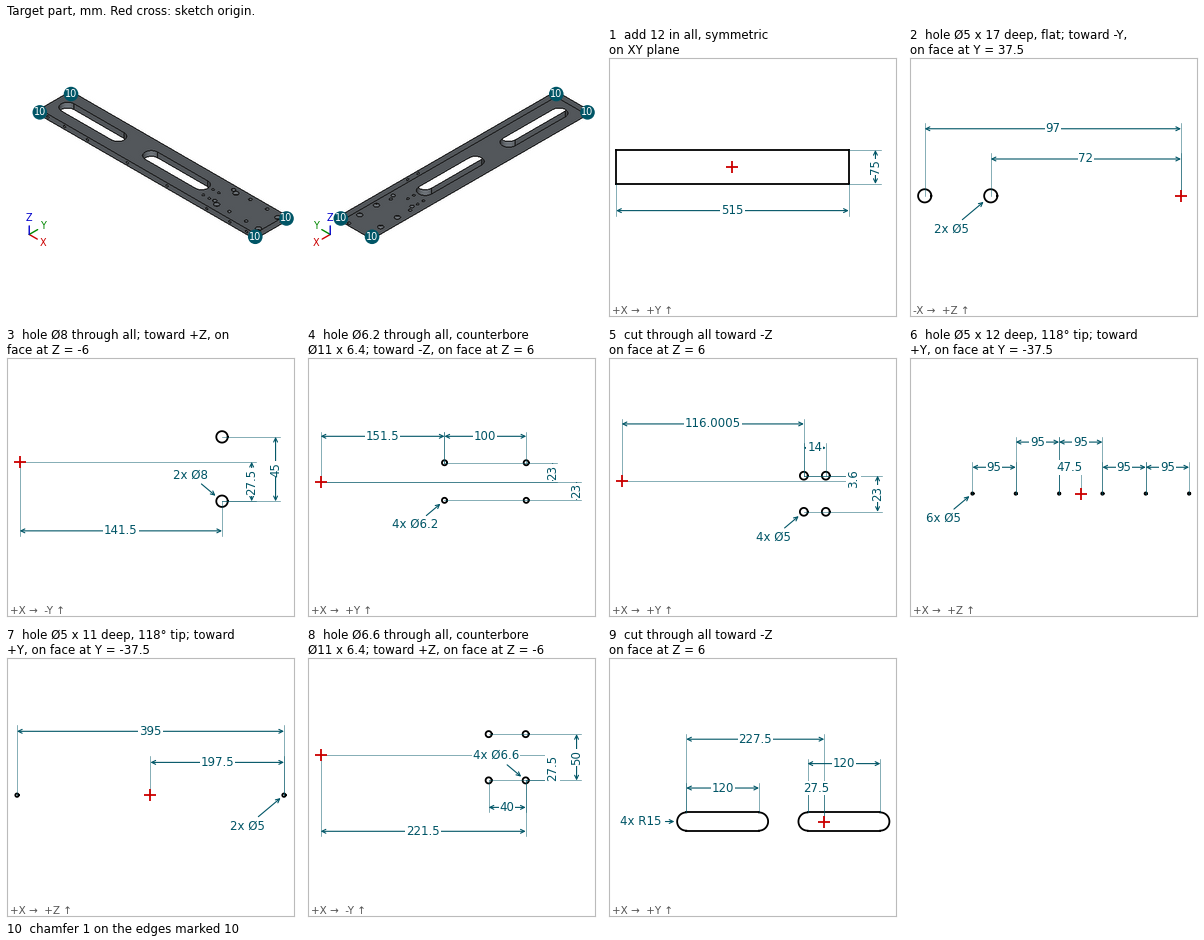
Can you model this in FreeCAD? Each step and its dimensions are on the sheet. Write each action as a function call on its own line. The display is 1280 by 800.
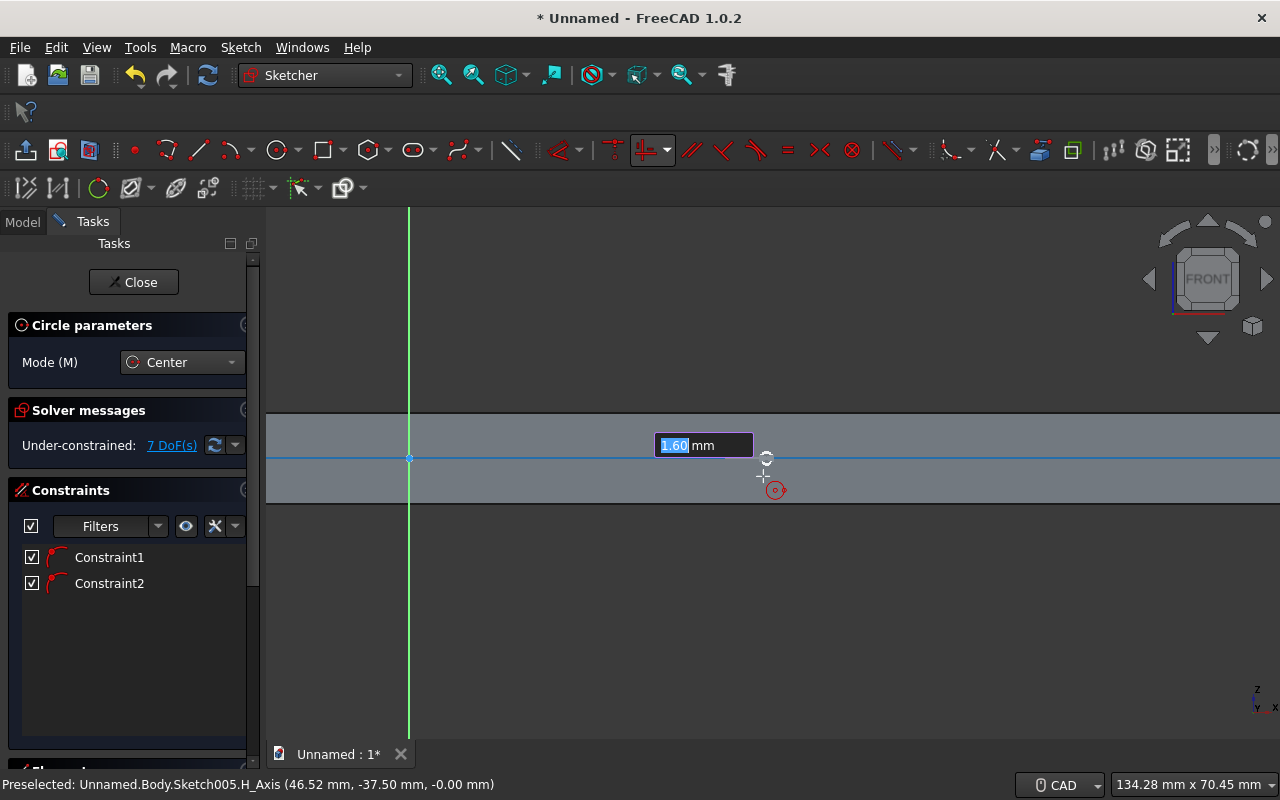
click(761, 476)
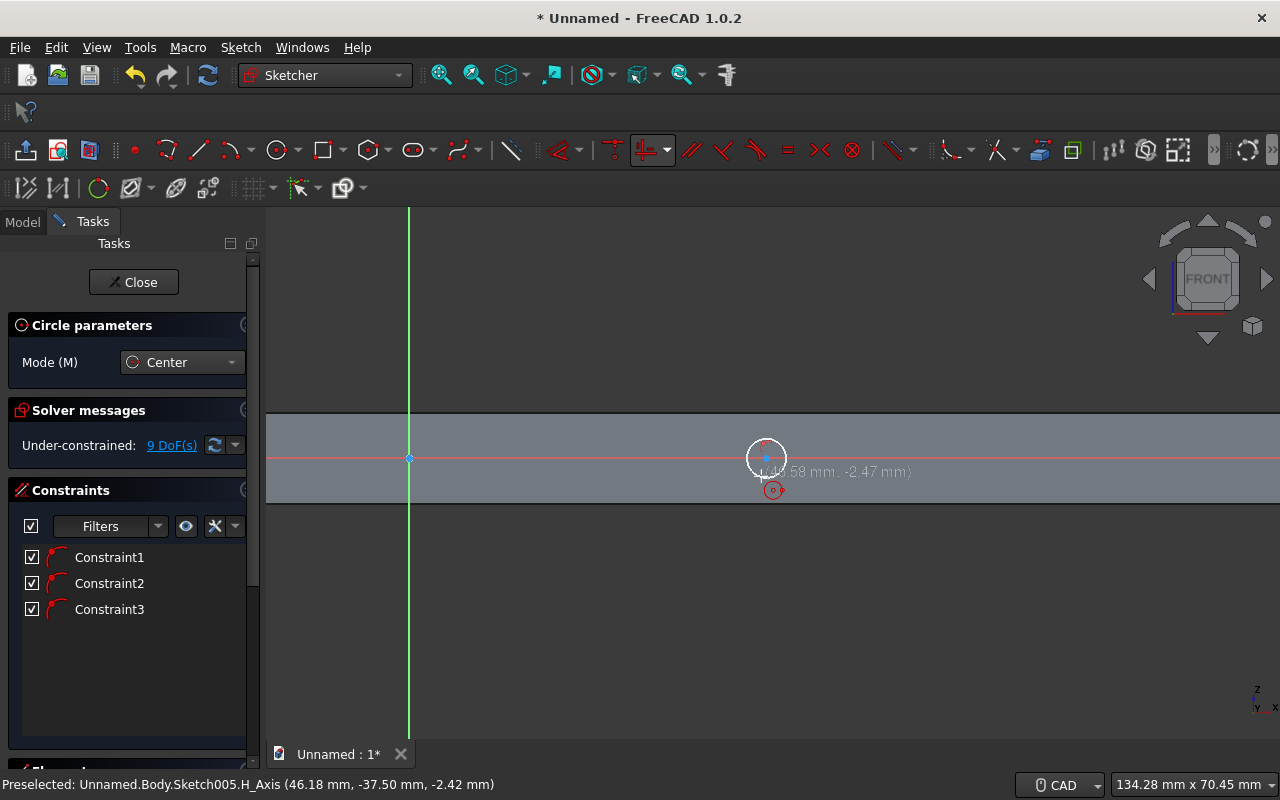
scroll(763, 476, down, 9)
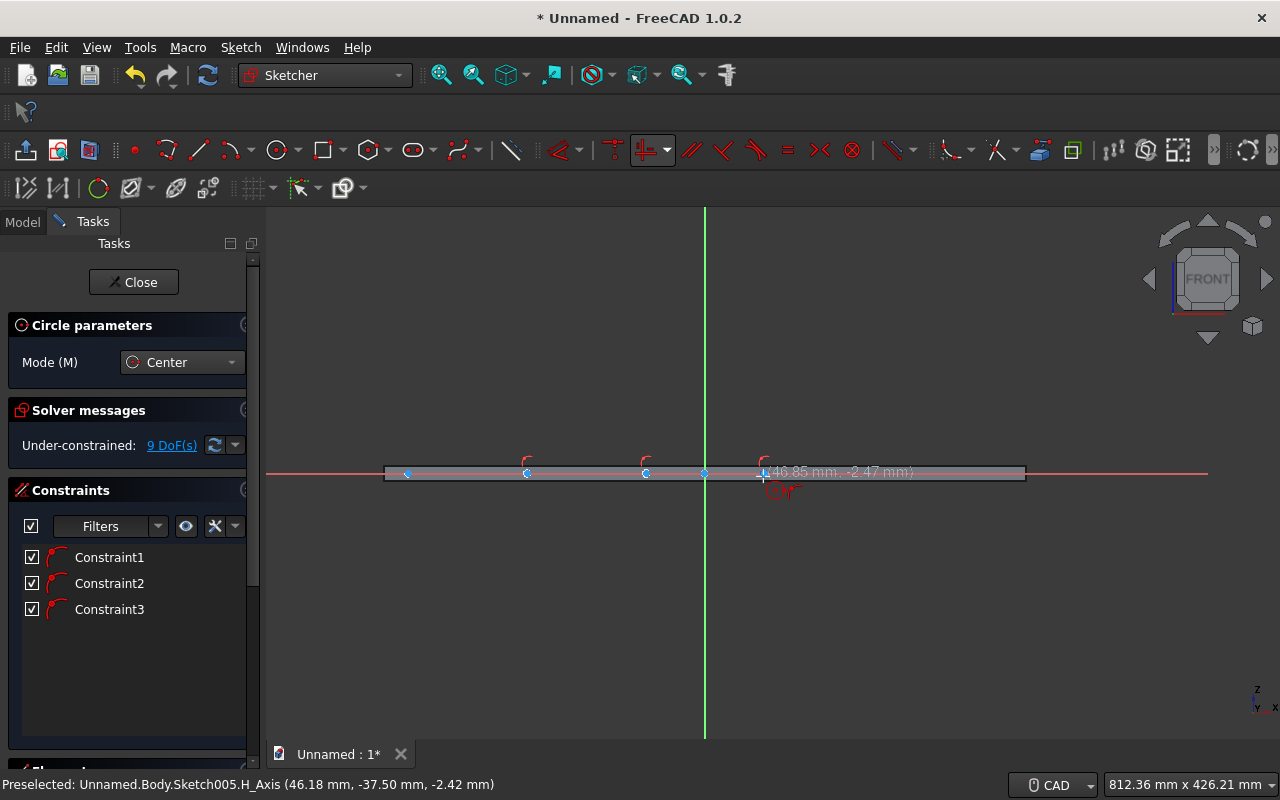
scroll(883, 473, up, 10)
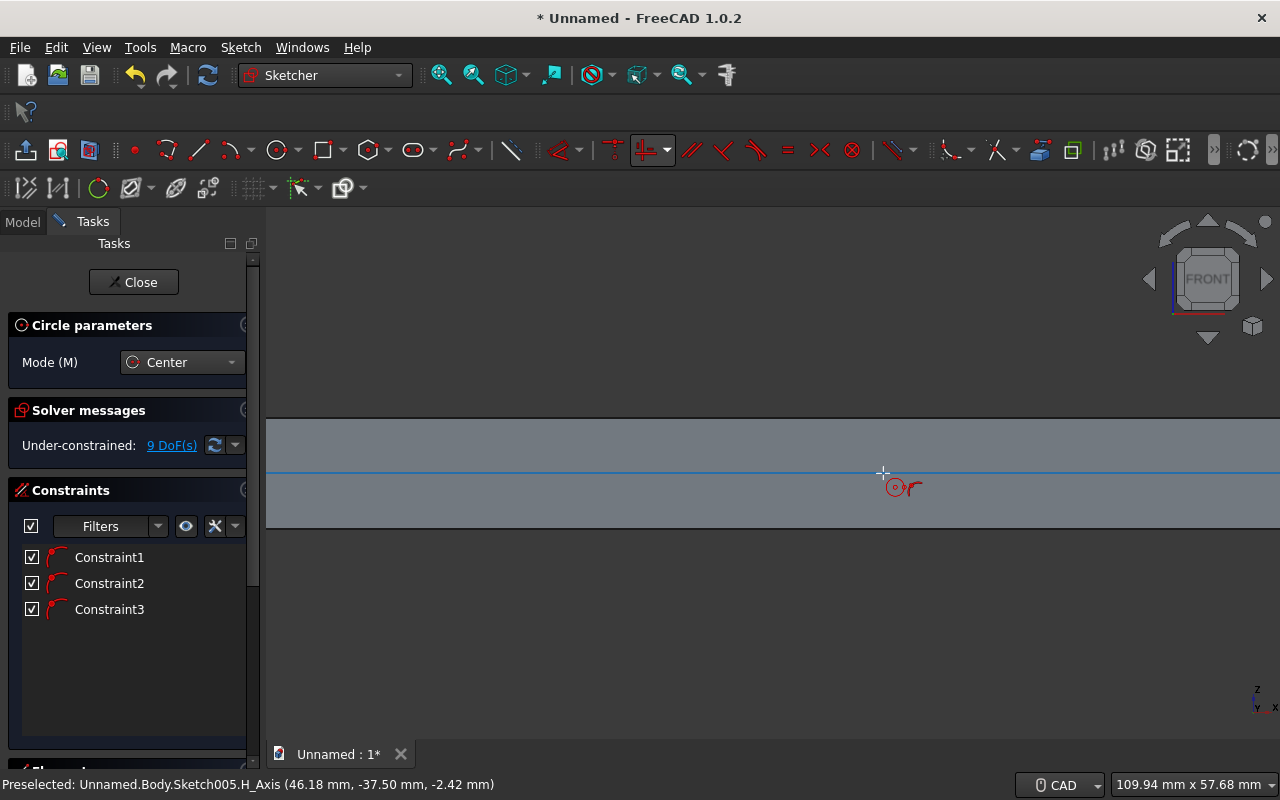
scroll(883, 473, down, 10)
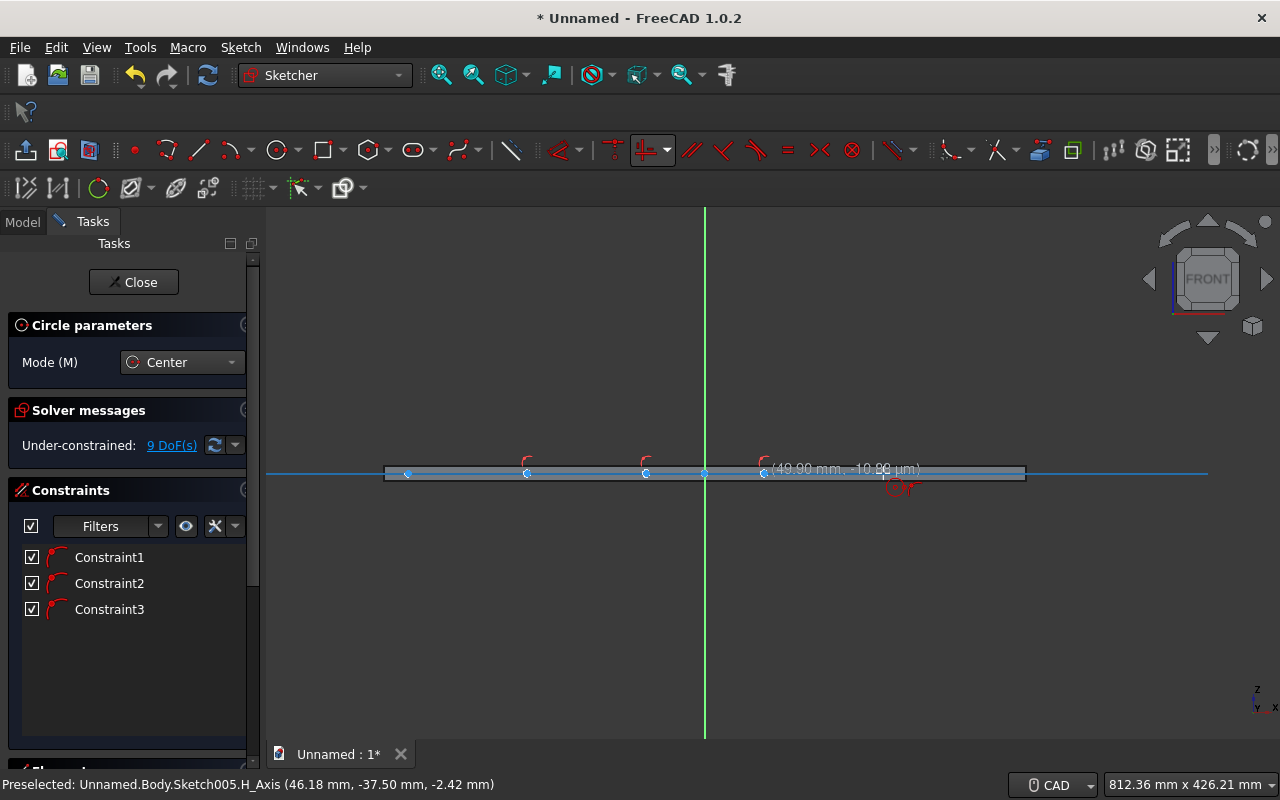
click(883, 473)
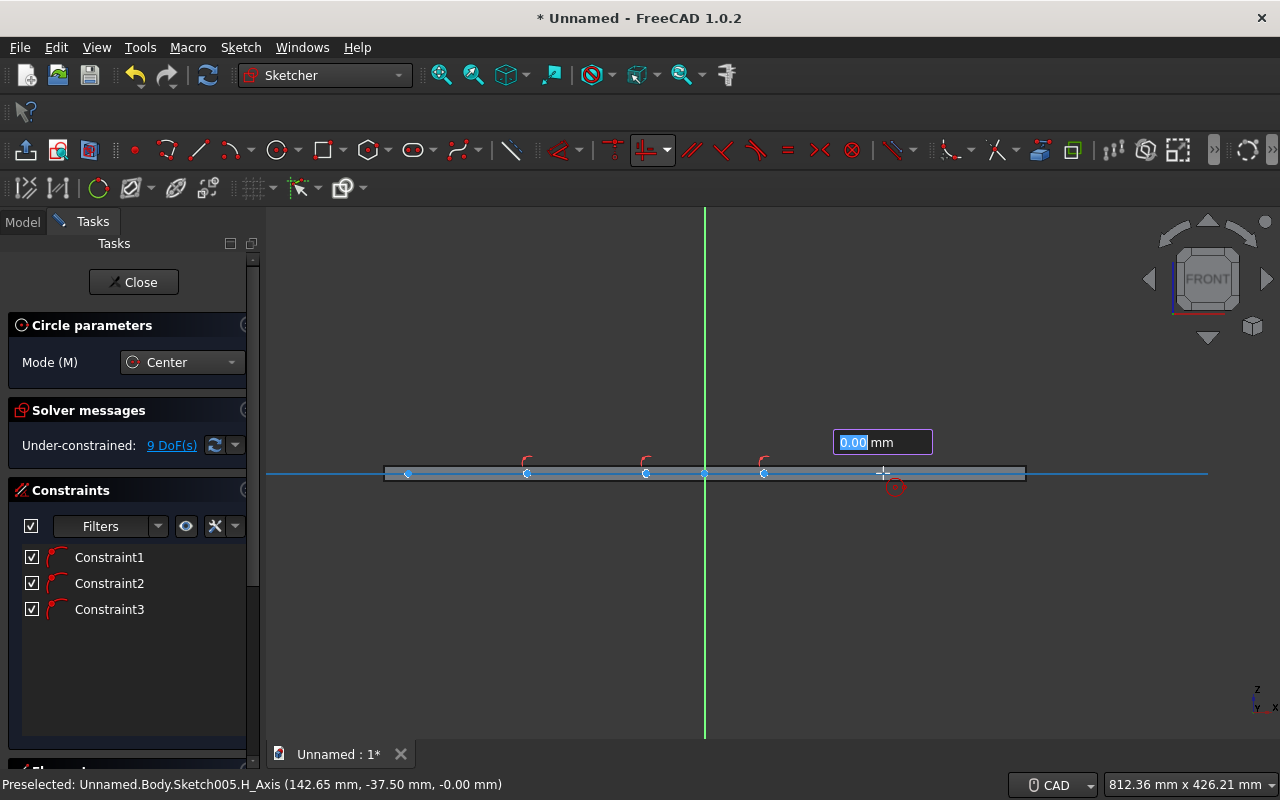
scroll(882, 476, up, 9)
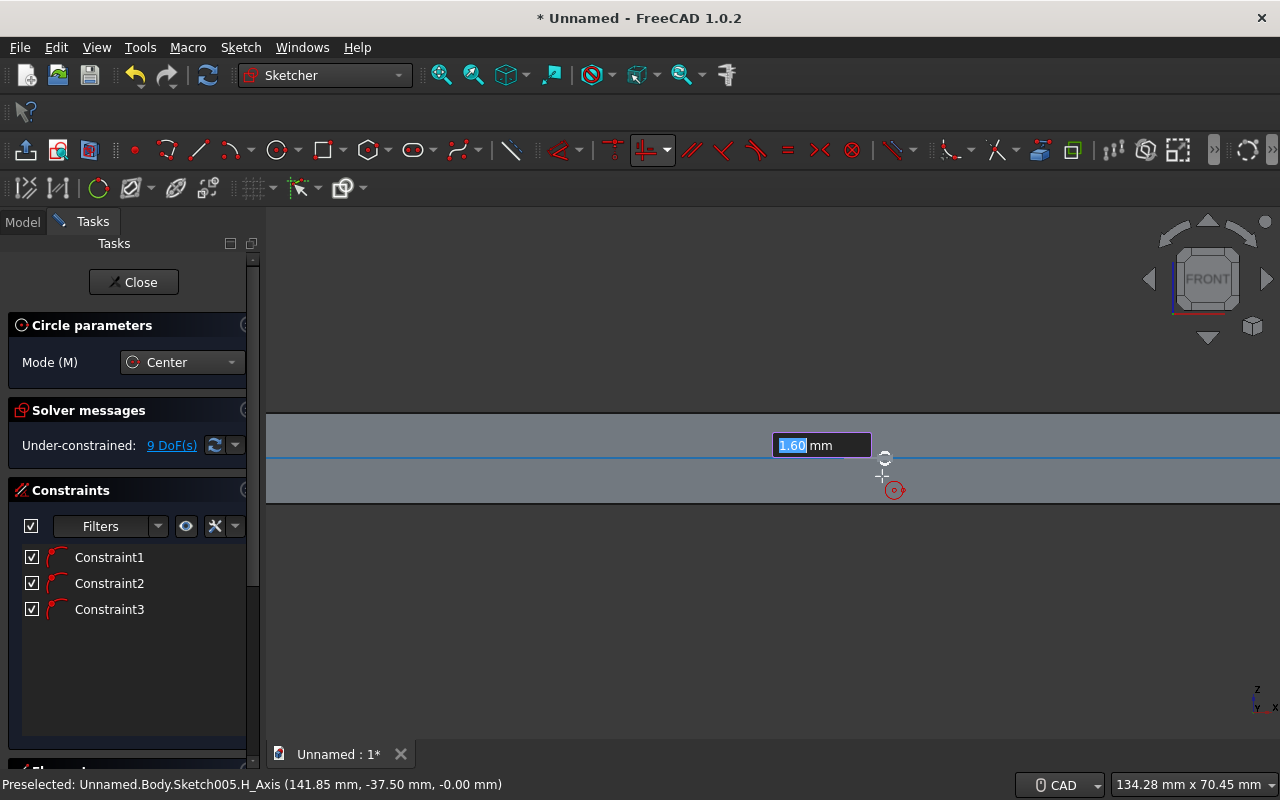
click(877, 476)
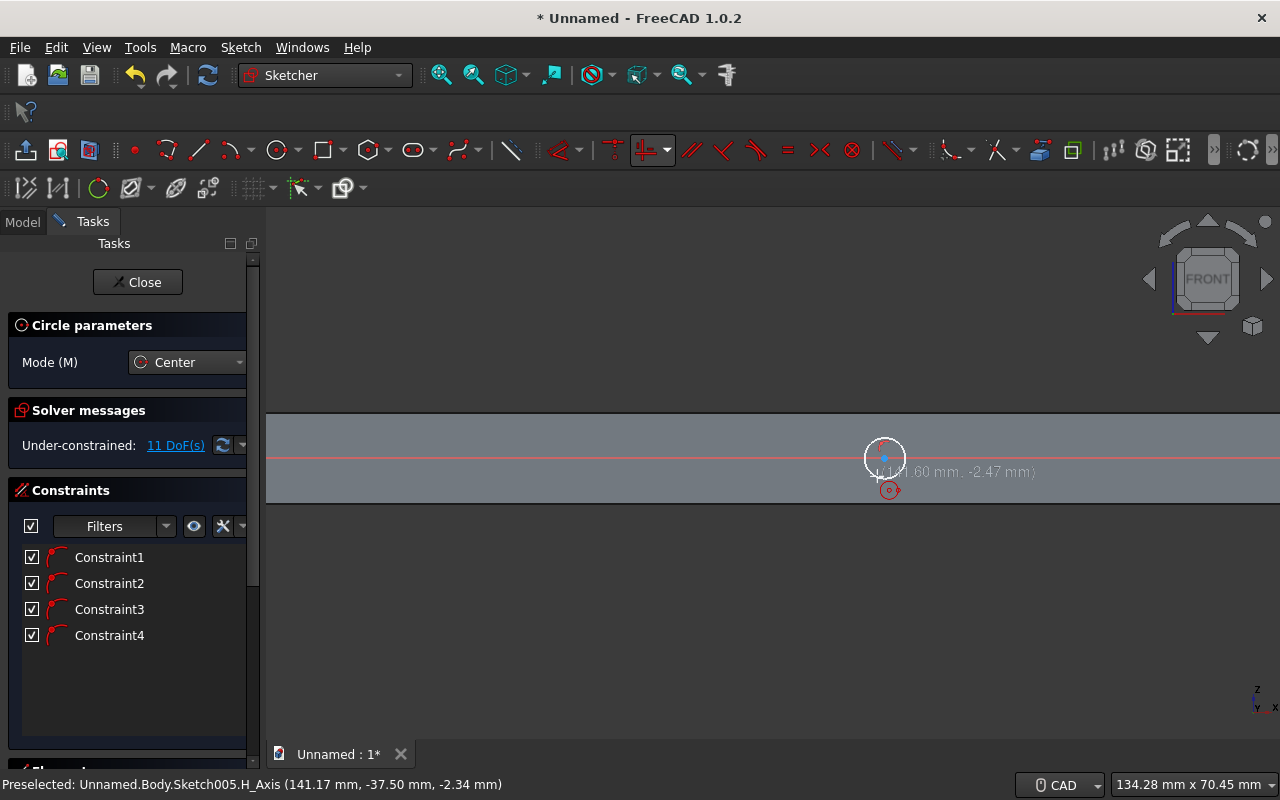
scroll(882, 476, down, 9)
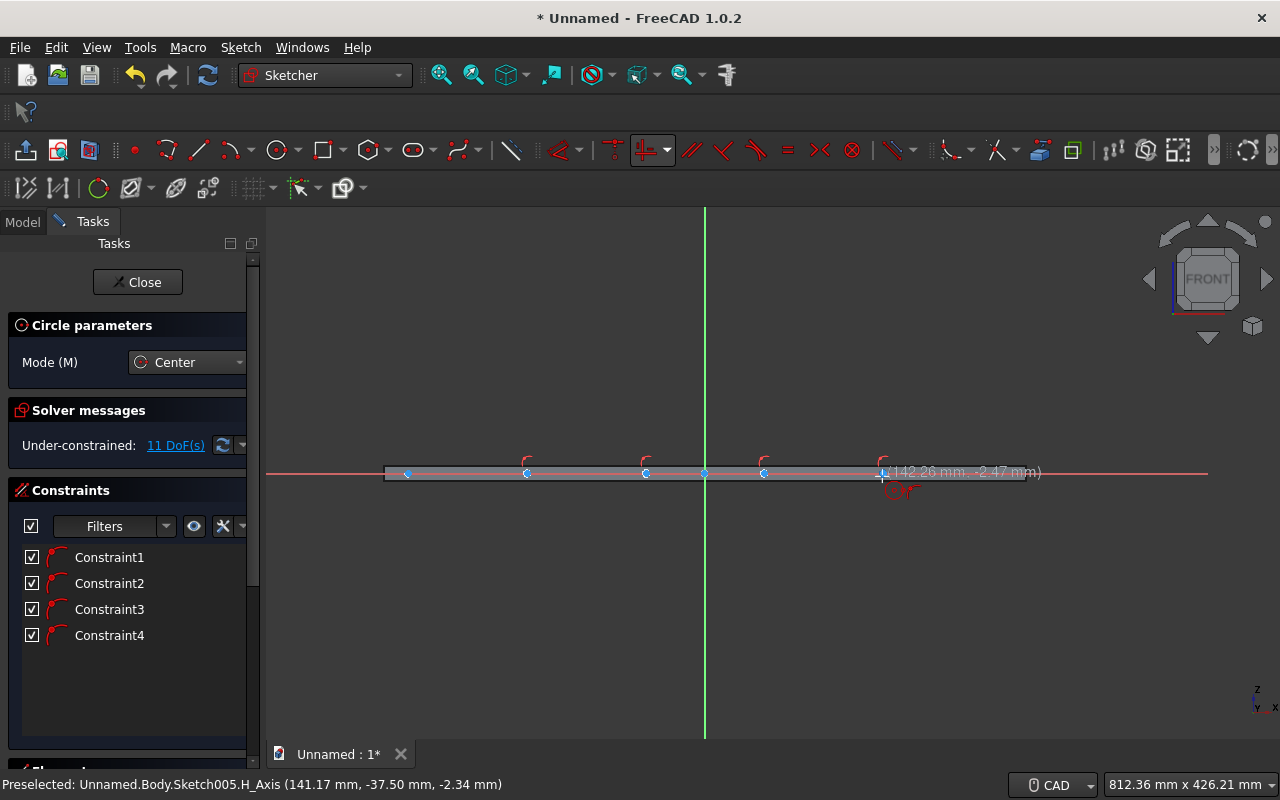
scroll(1001, 473, up, 10)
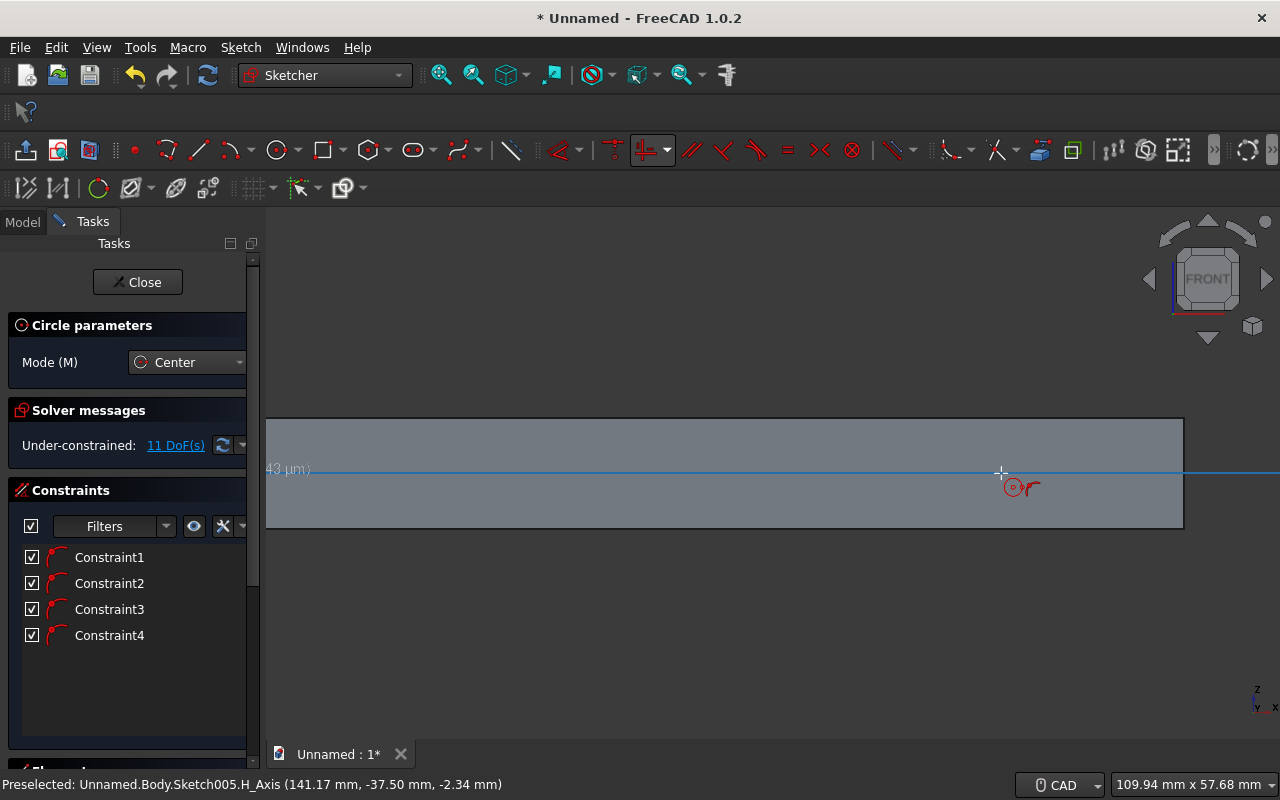
scroll(1001, 473, down, 10)